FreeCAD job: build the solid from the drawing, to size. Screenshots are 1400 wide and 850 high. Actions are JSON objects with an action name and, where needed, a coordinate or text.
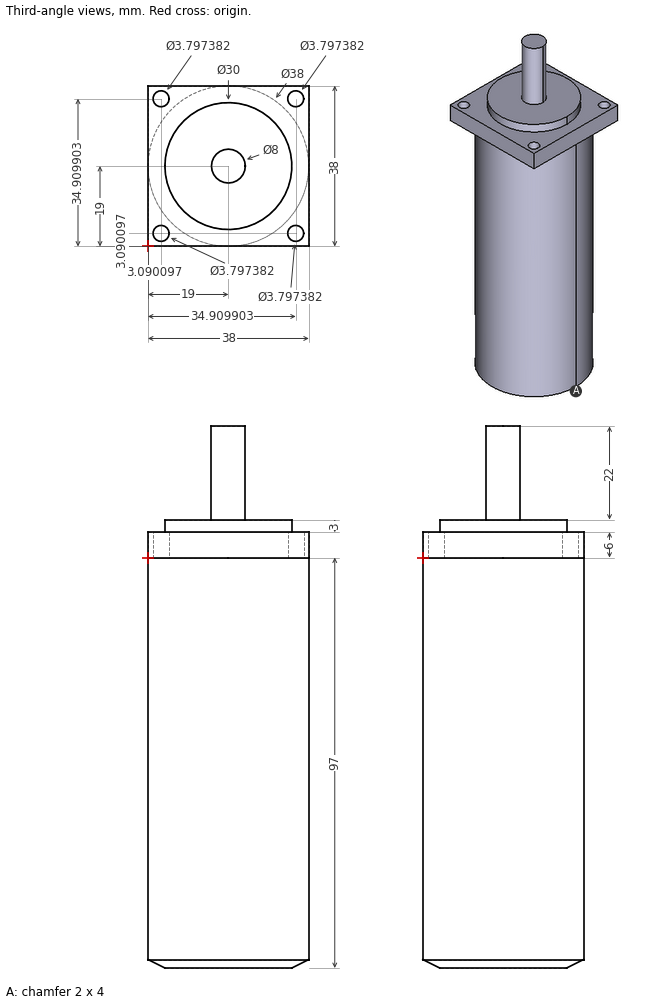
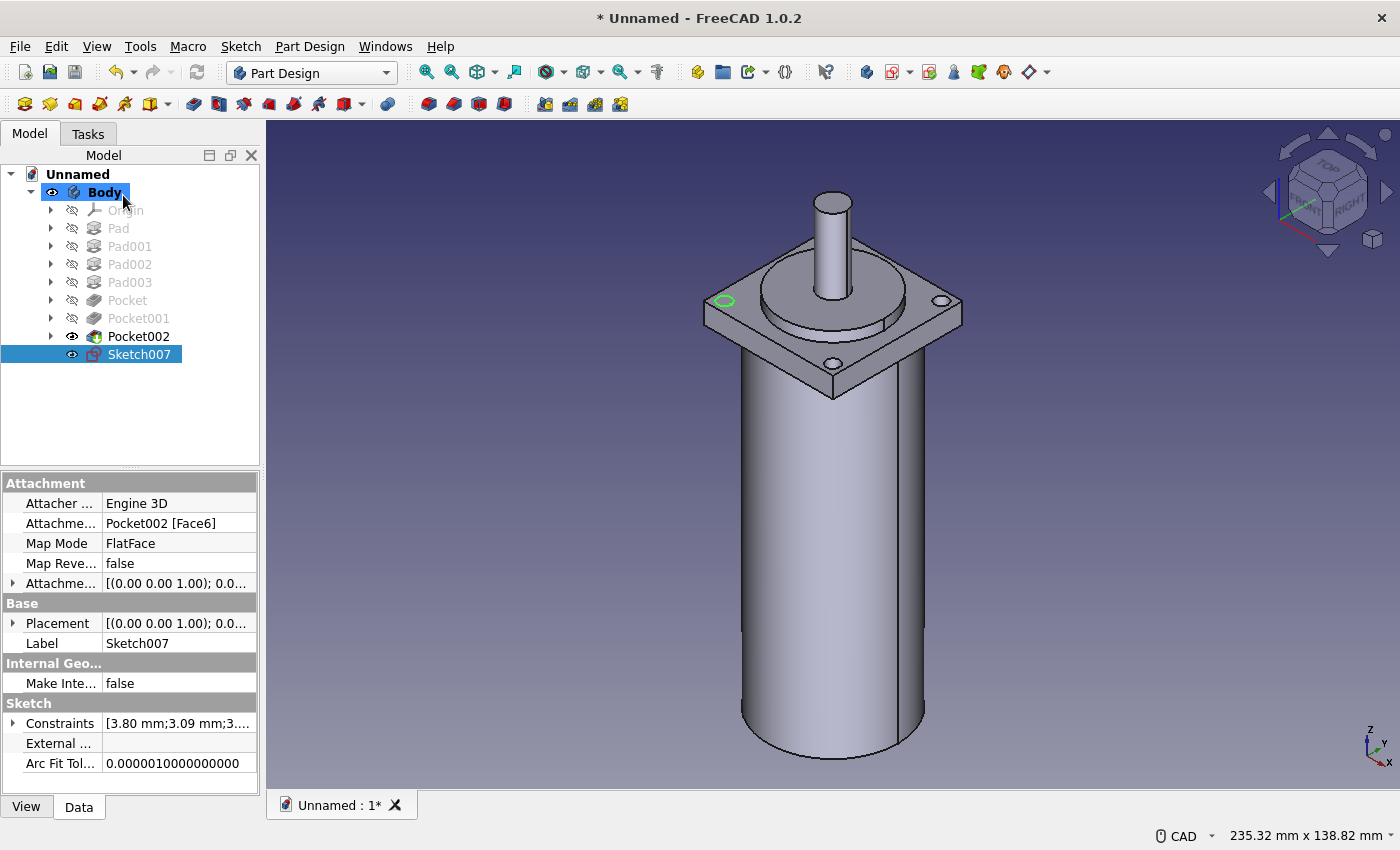
{"action": "left_click", "coordinate": [194, 104]}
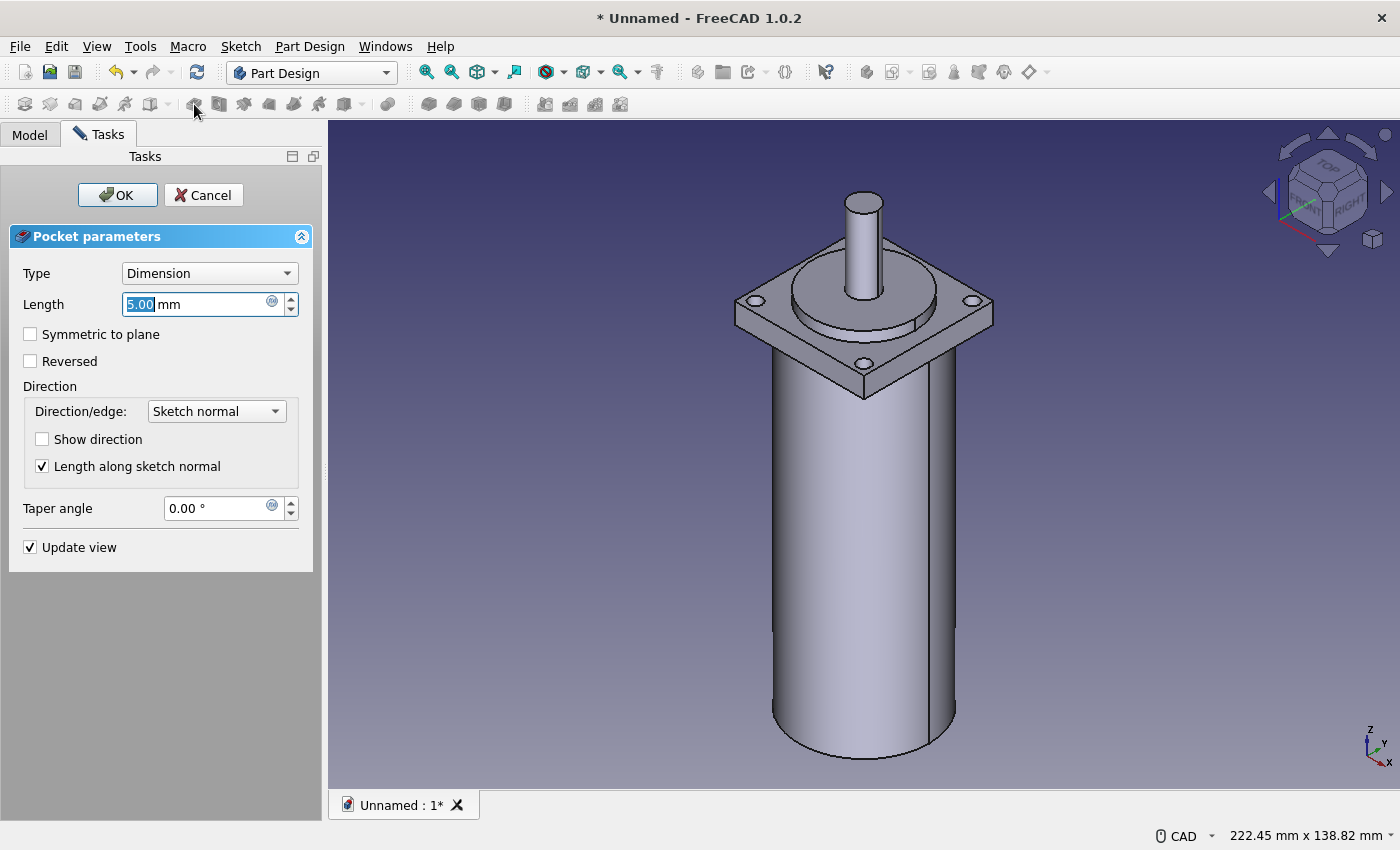
{"action": "left_click", "coordinate": [210, 274]}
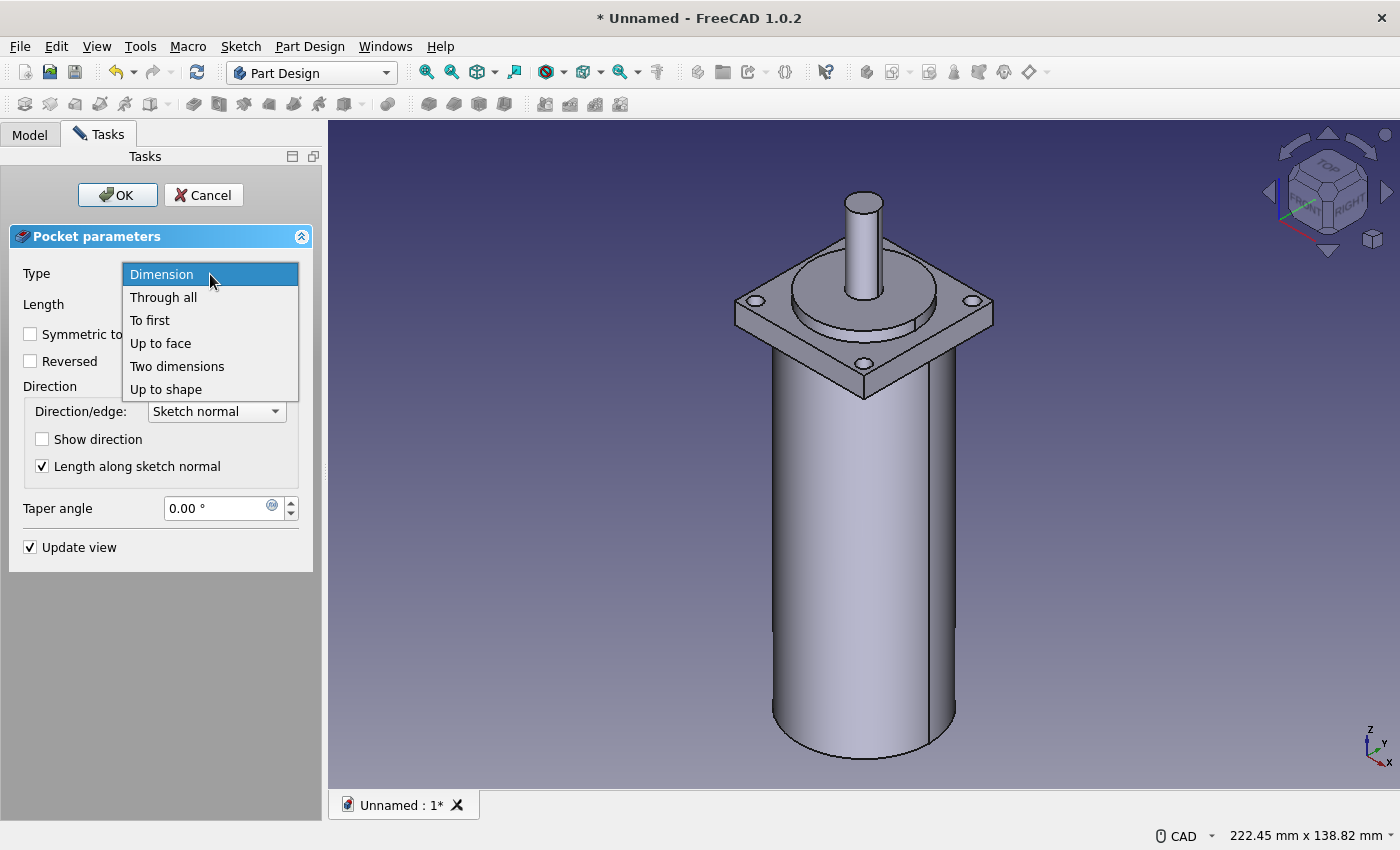
{"action": "left_click", "coordinate": [208, 320]}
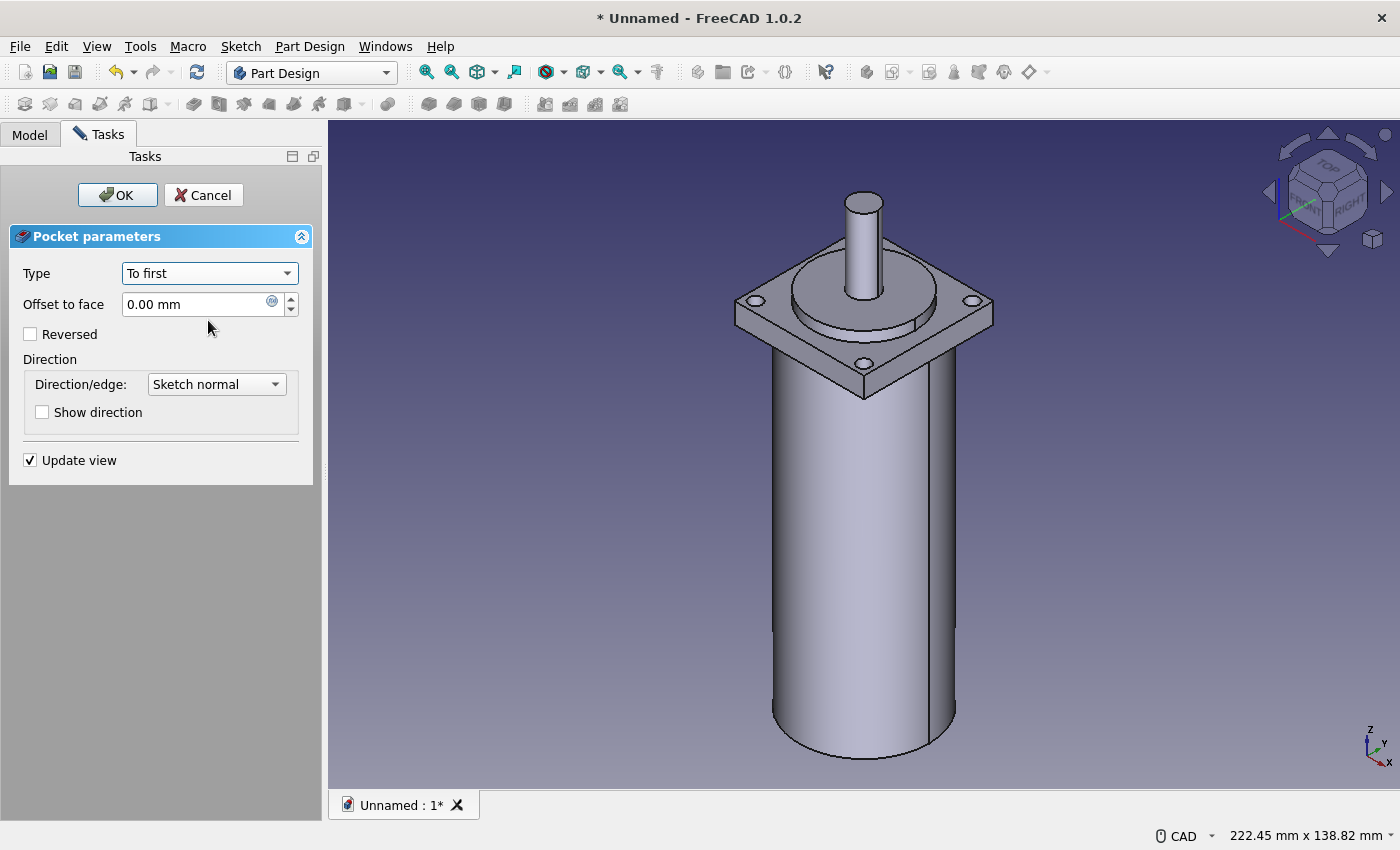
{"action": "left_click", "coordinate": [118, 195]}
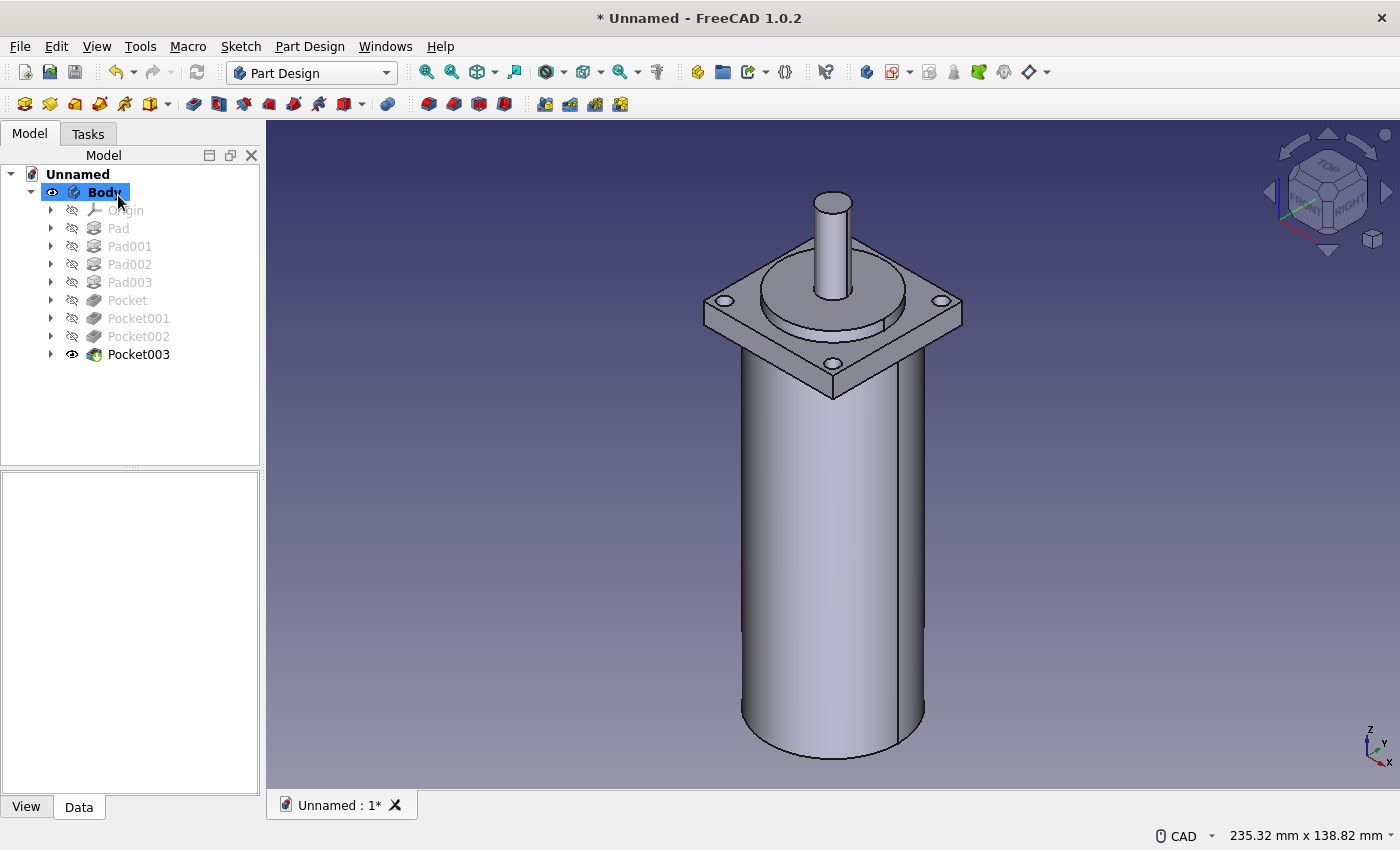
{"action": "key", "text": "2"}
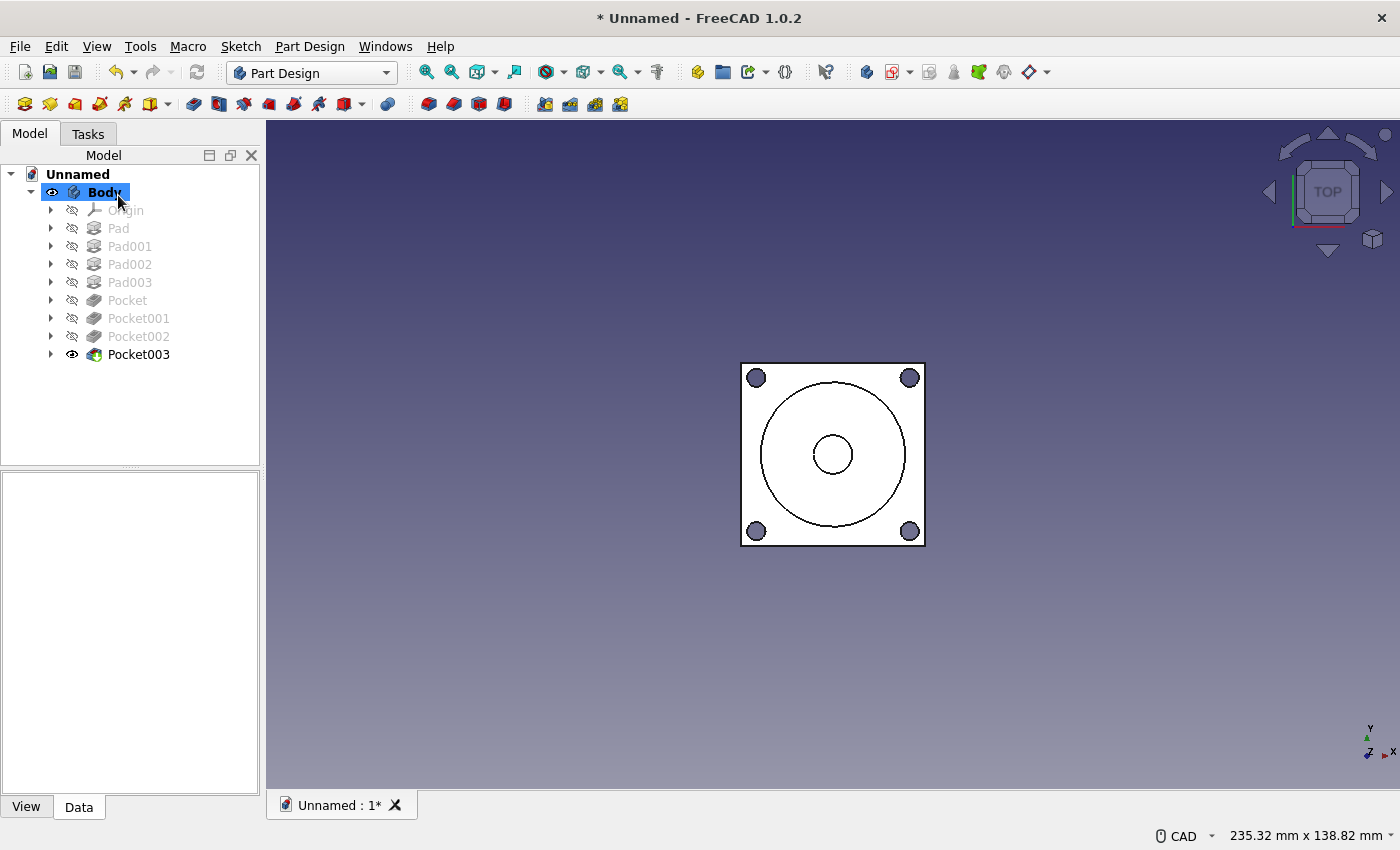
{"action": "left_click", "coordinate": [427, 72]}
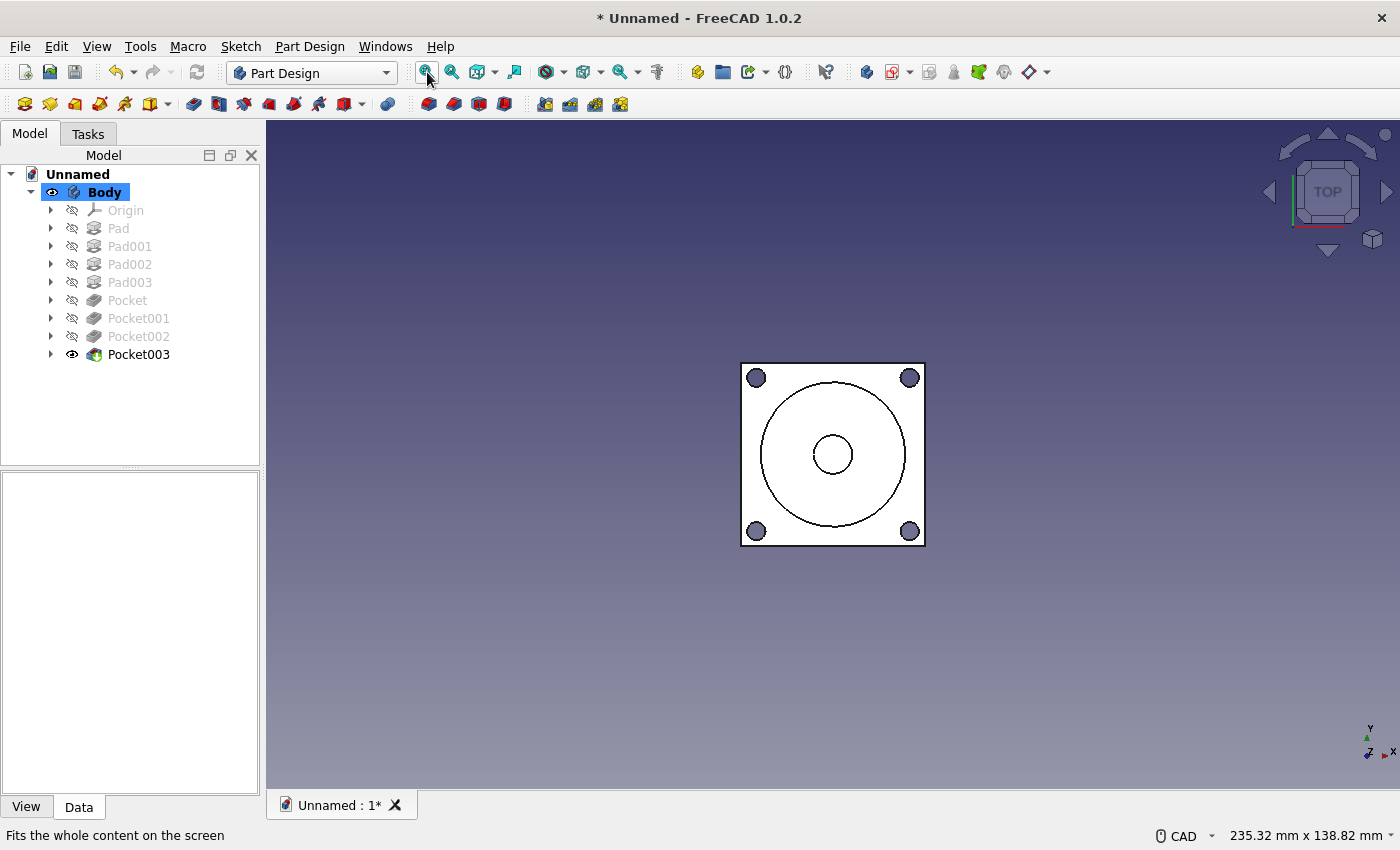
{"action": "key", "text": "0"}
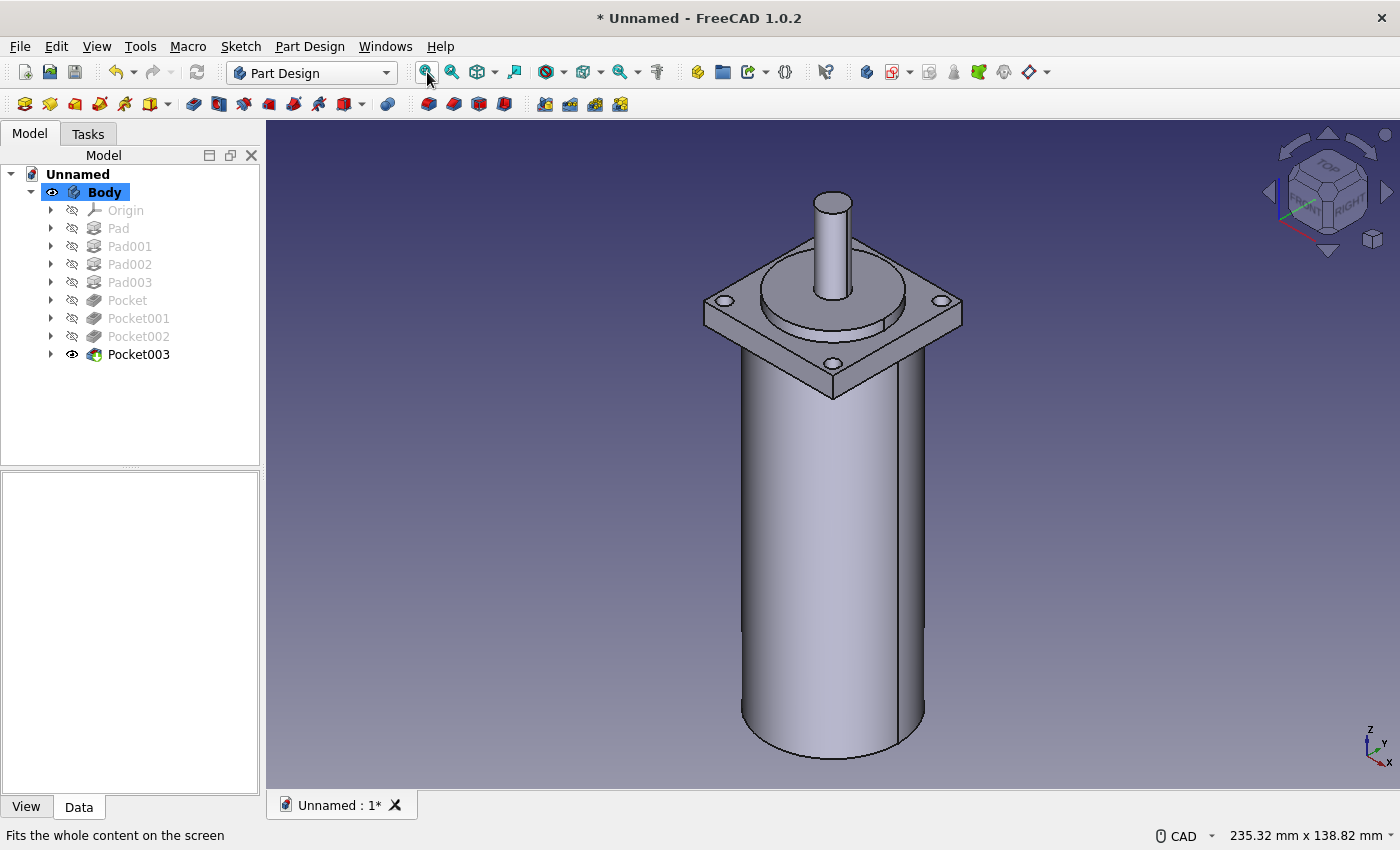
{"action": "key", "text": "1"}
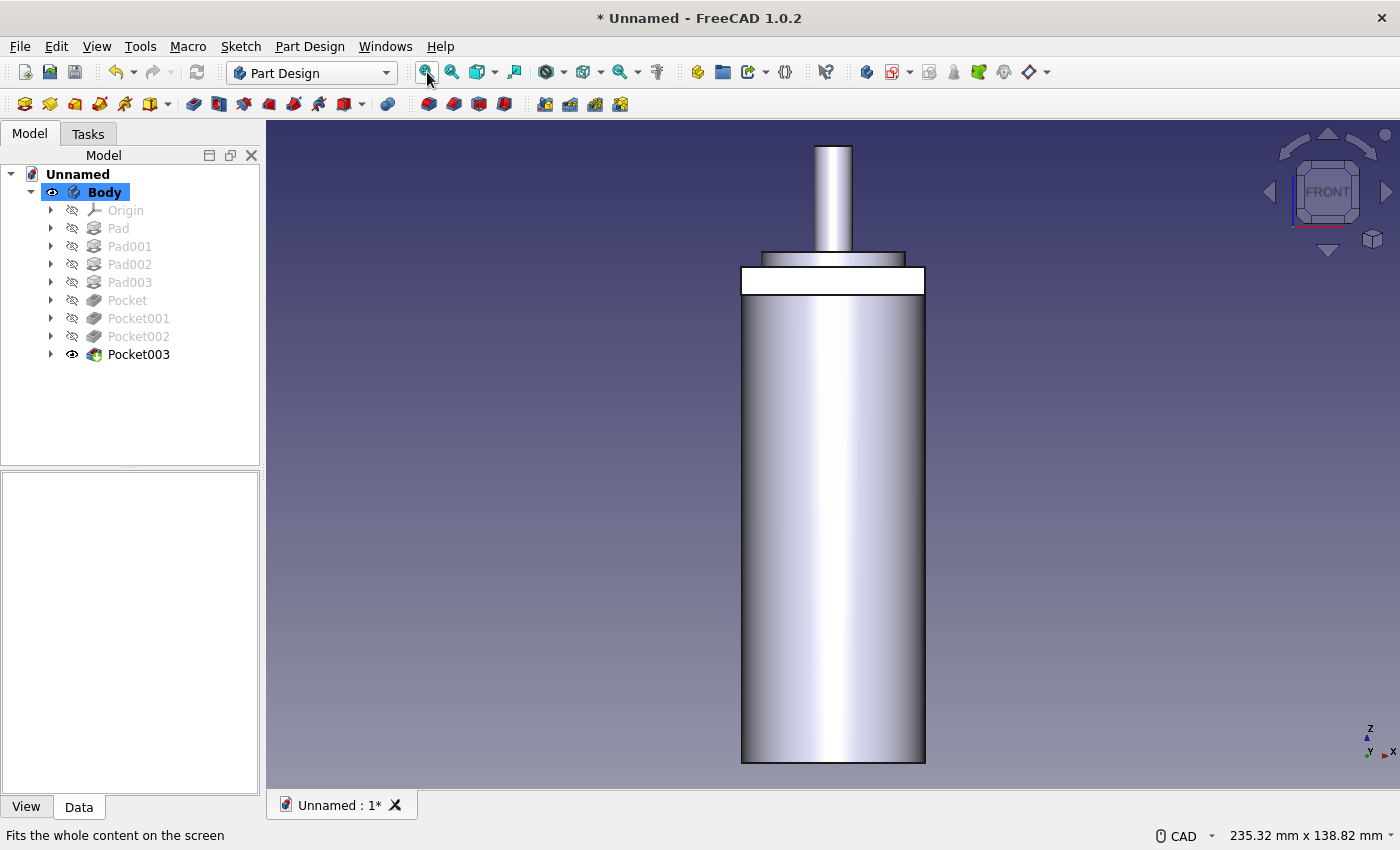
{"action": "key", "text": "3"}